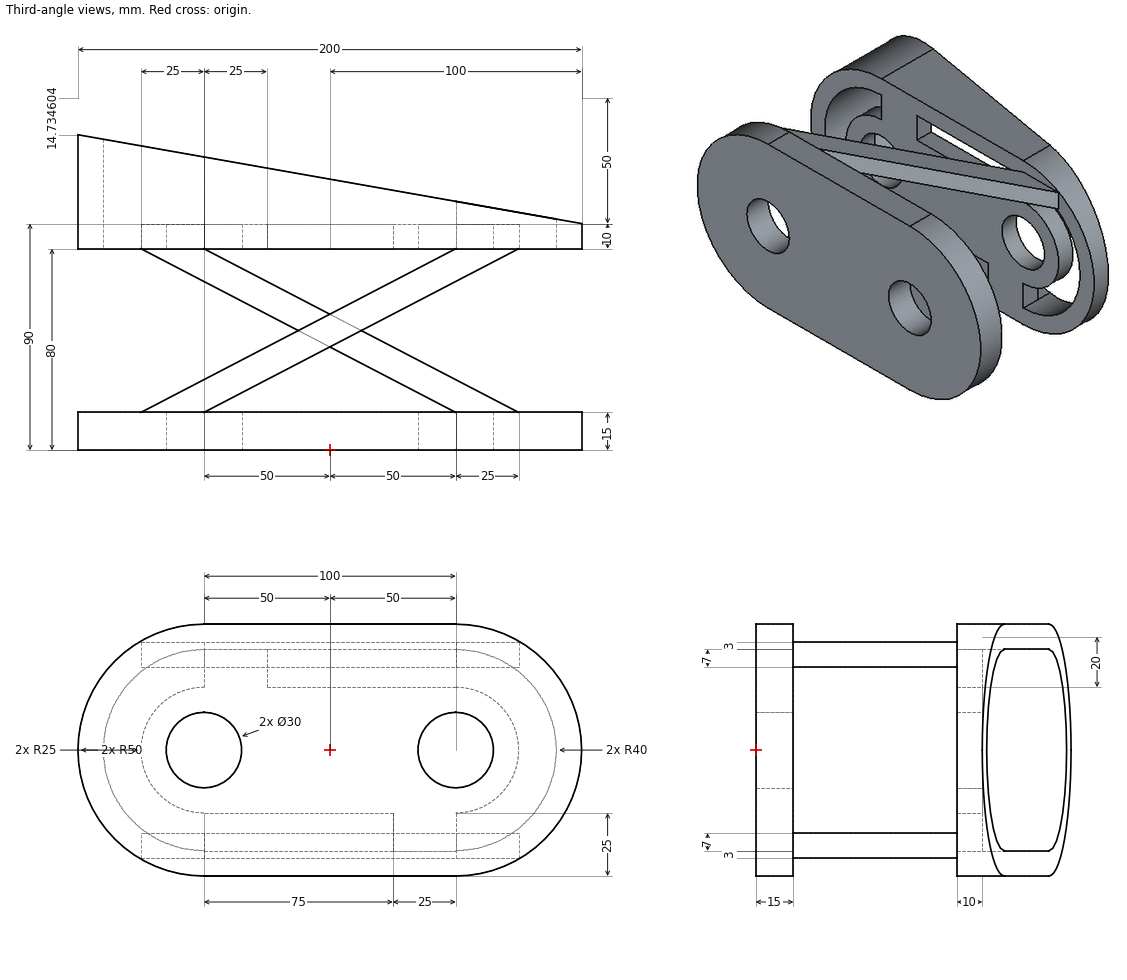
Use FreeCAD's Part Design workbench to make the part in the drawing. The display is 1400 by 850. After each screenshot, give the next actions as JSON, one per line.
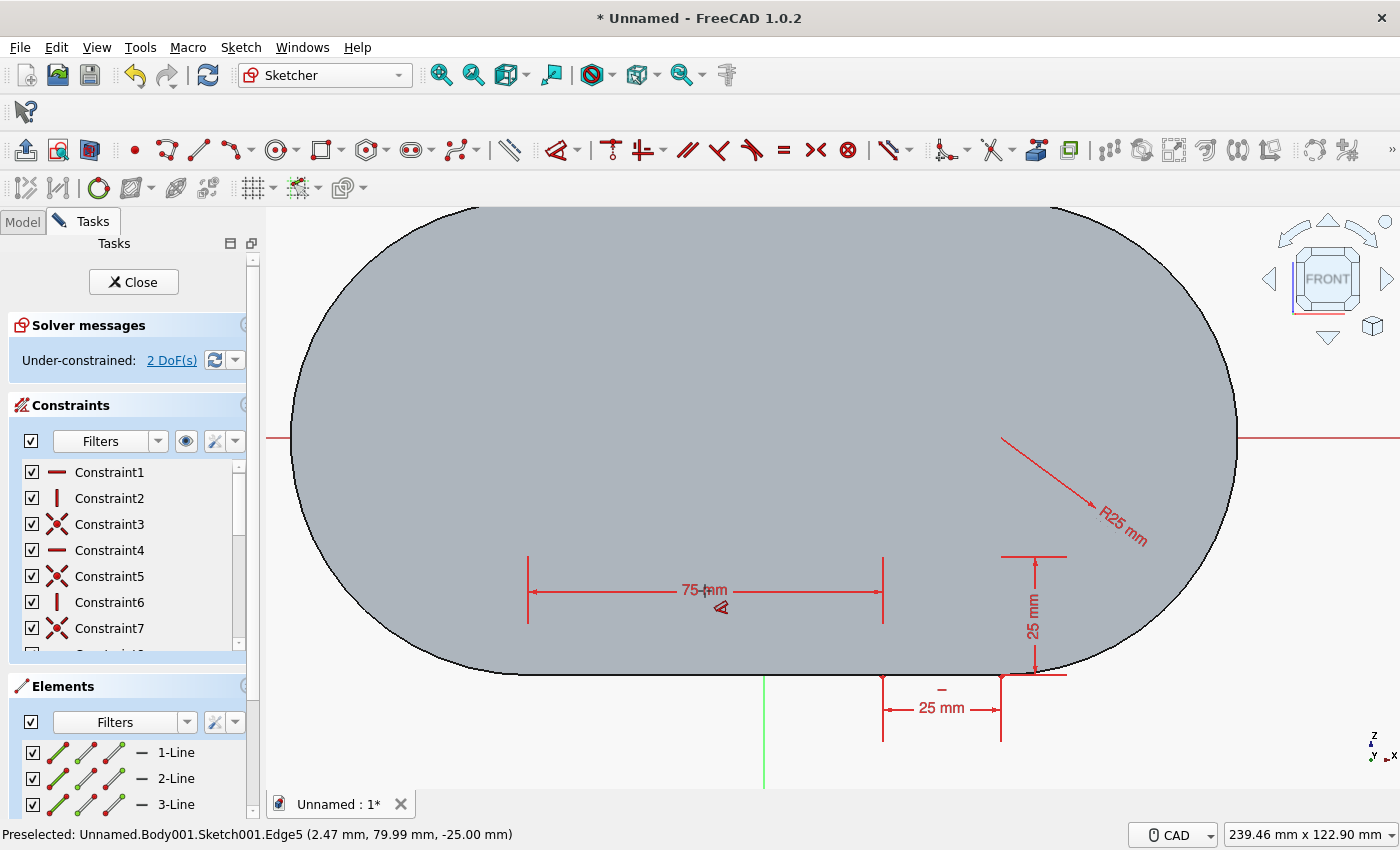
{"action": "left_click", "coordinate": [670, 320]}
{"action": "left_click", "coordinate": [656, 286]}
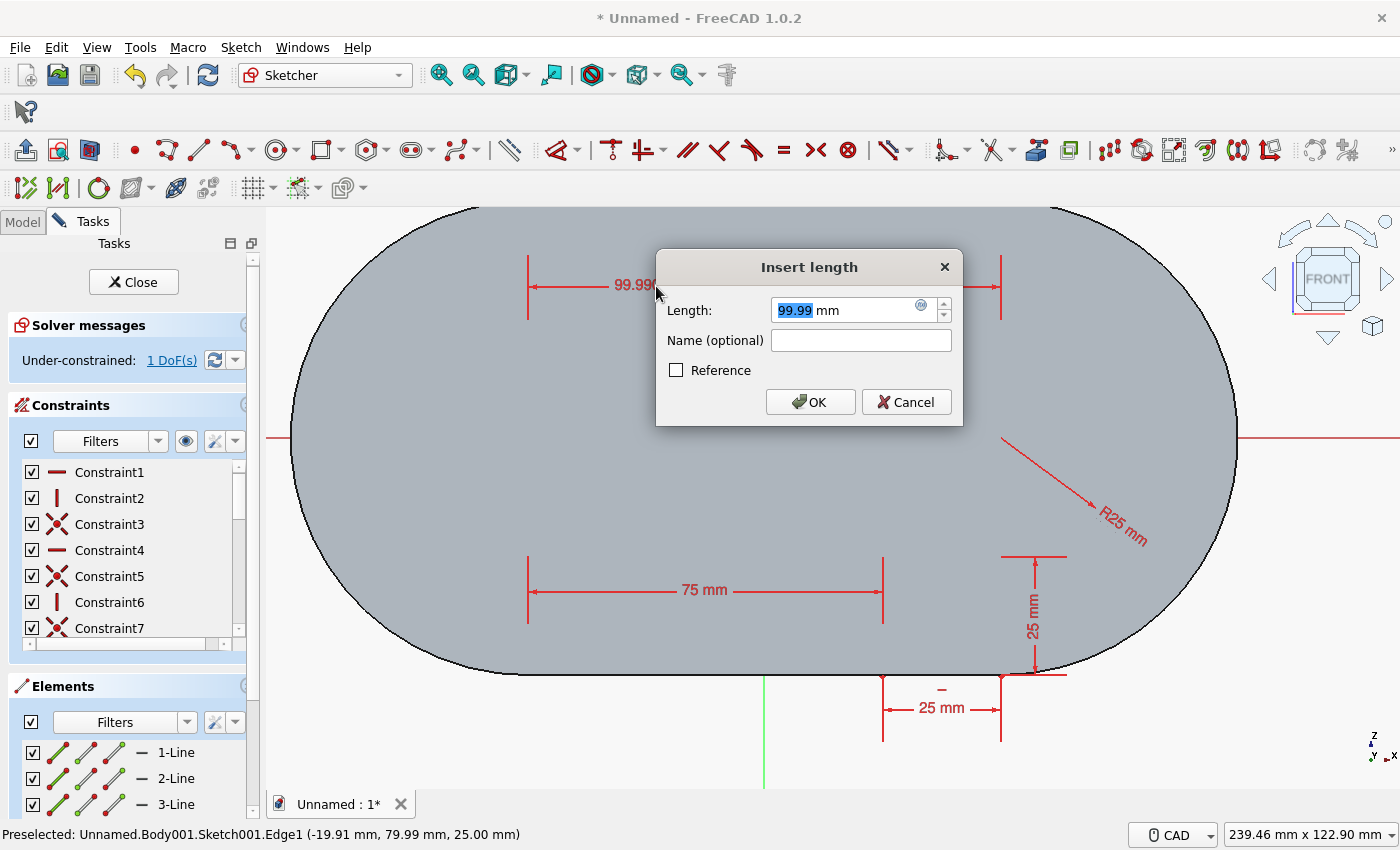
{"action": "type", "text": "100"}
{"action": "key", "text": "Return"}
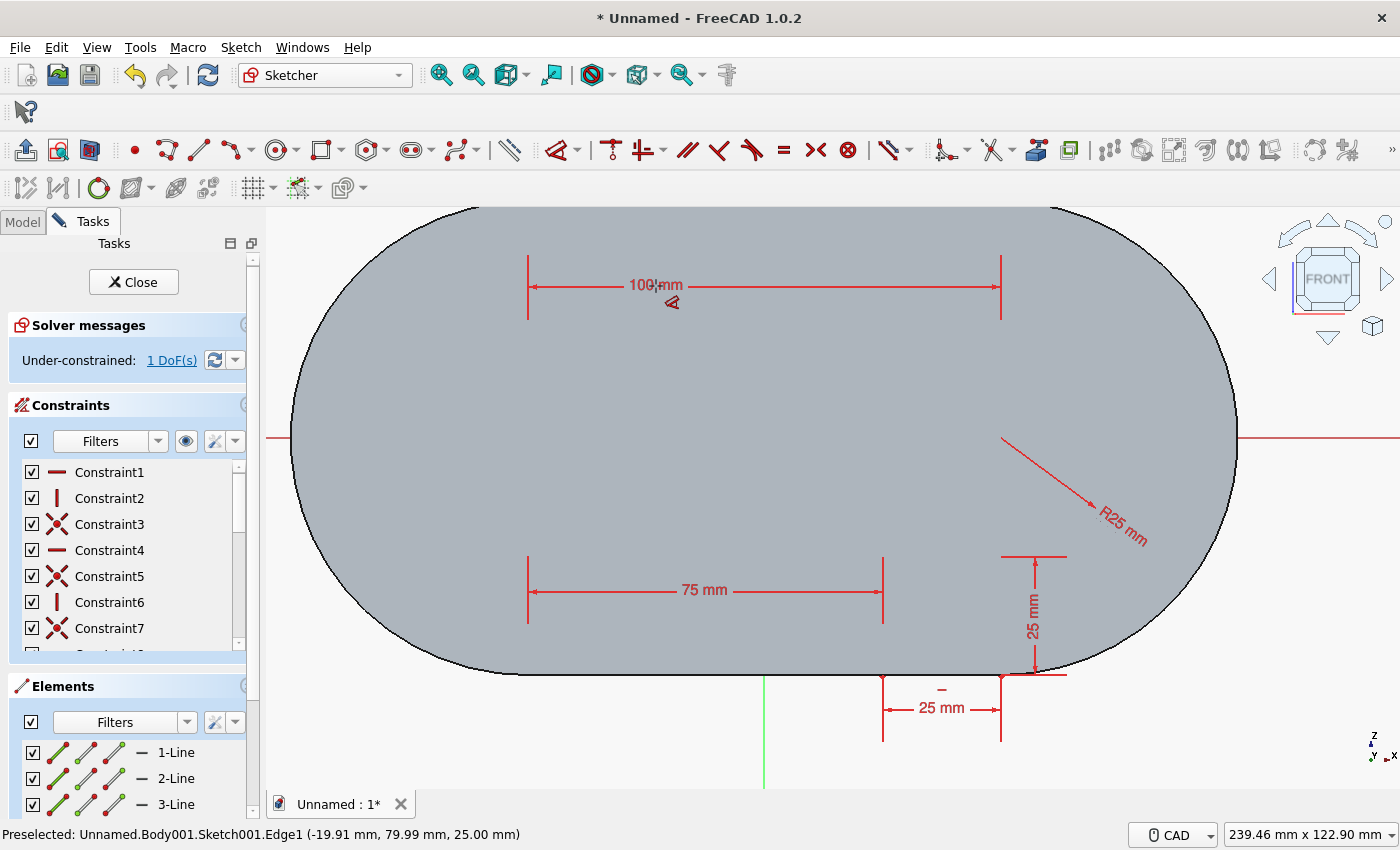
{"action": "left_click", "coordinate": [528, 320]}
{"action": "left_click", "coordinate": [563, 286]}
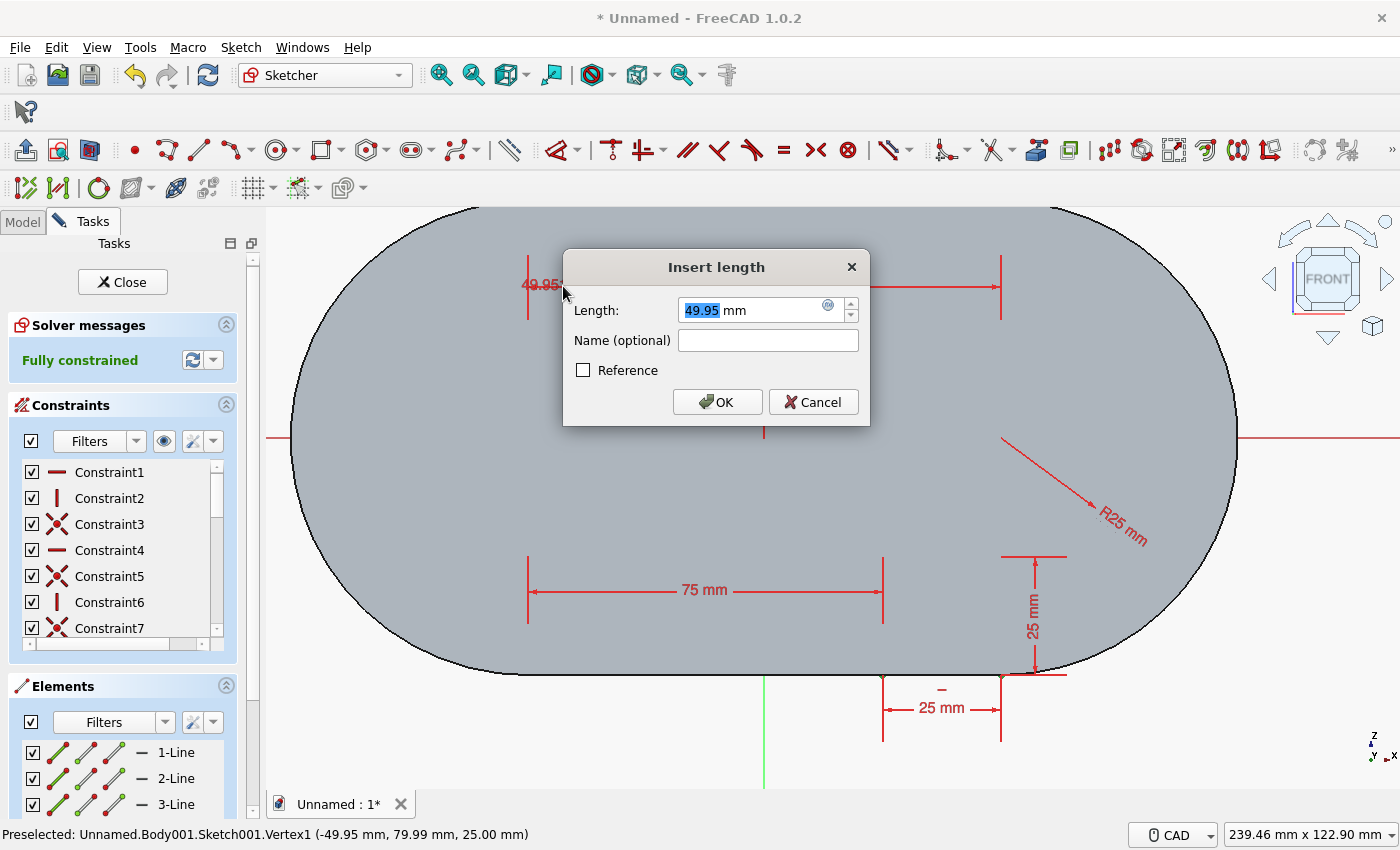
{"action": "type", "text": "50"}
{"action": "key", "text": "Return"}
{"action": "key", "text": "Escape"}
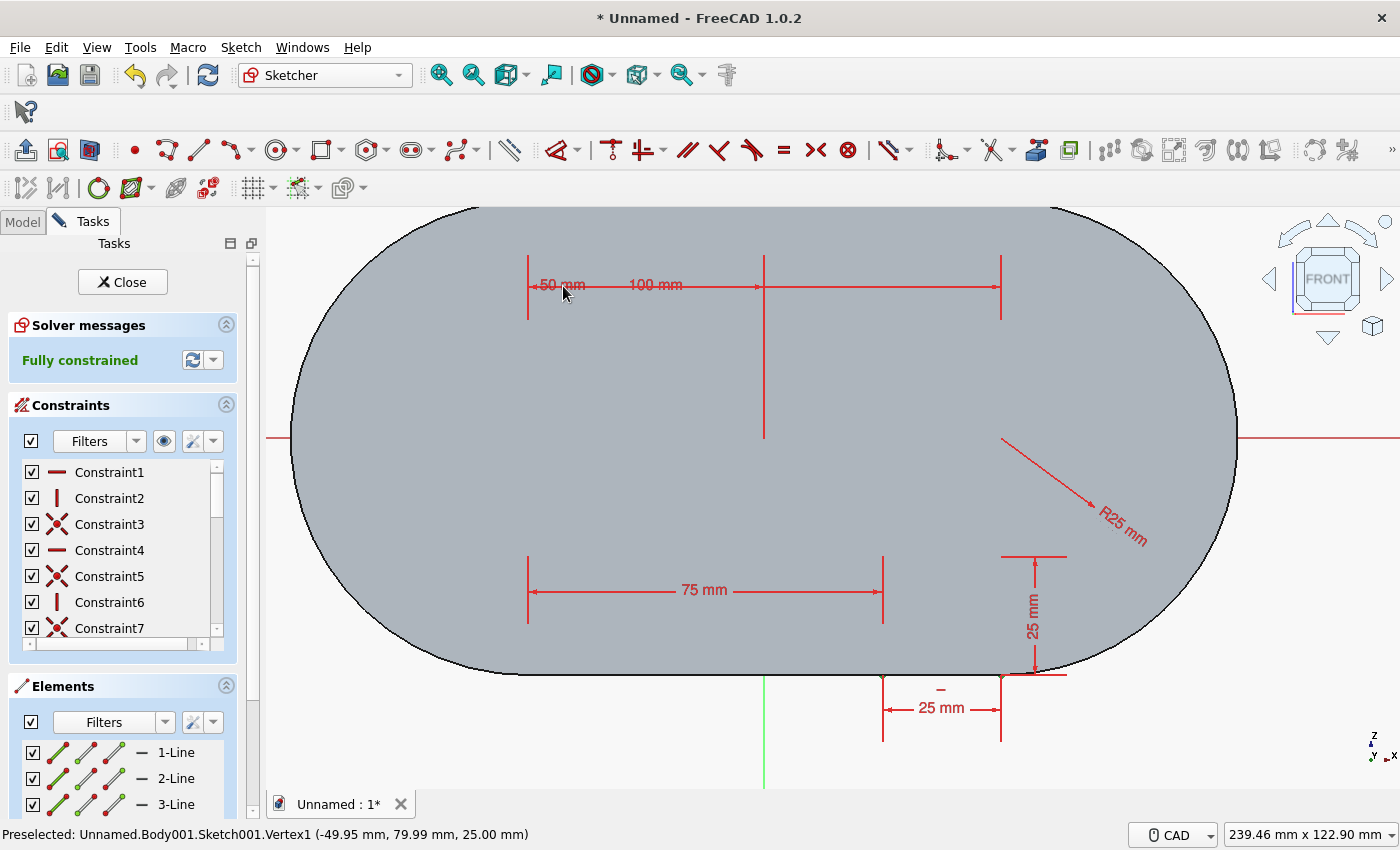
{"action": "left_click", "coordinate": [123, 282]}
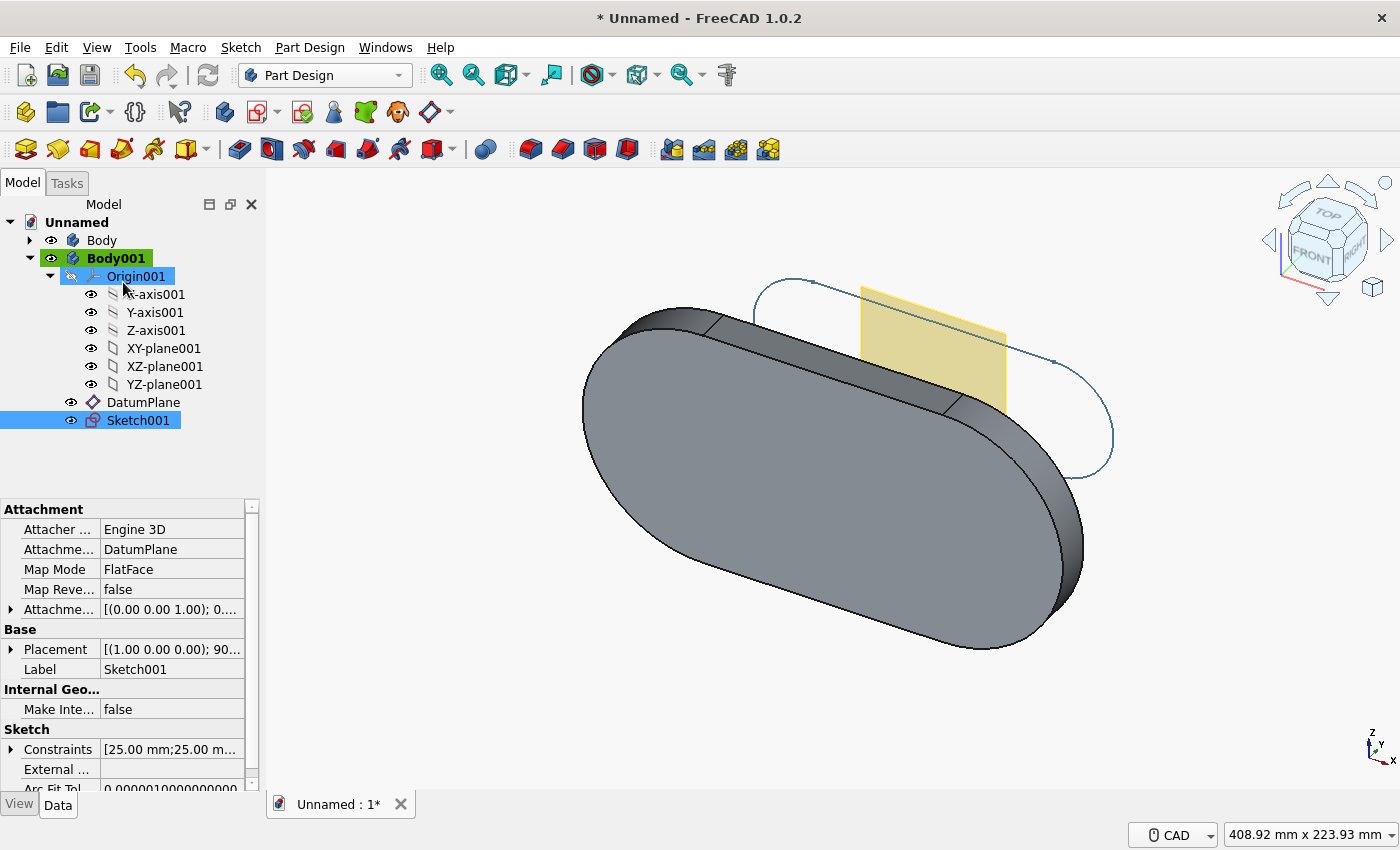
{"action": "left_click", "coordinate": [26, 150]}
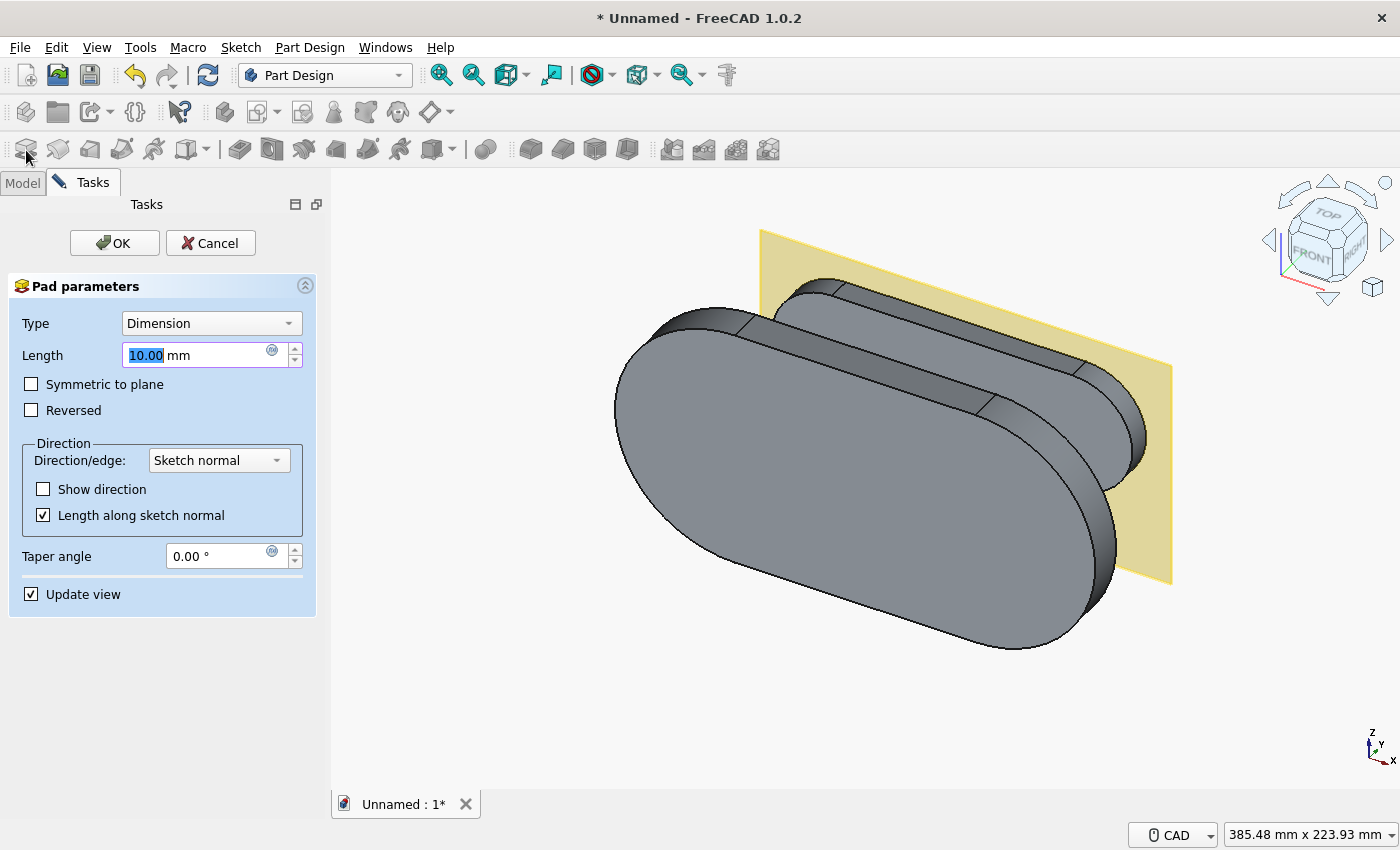
{"action": "type", "text": "10"}
{"action": "key", "text": "Tab"}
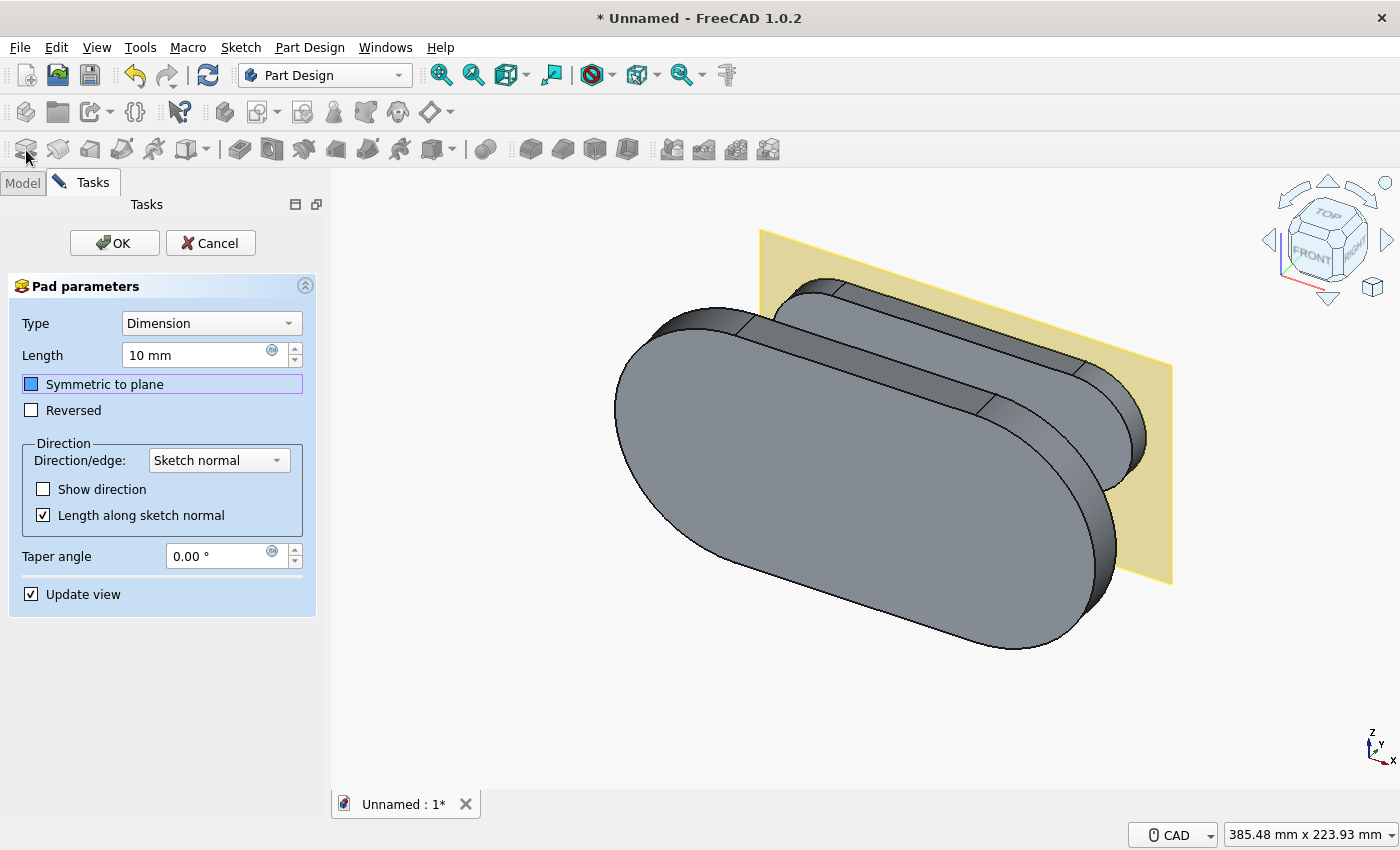
{"action": "left_click", "coordinate": [30, 410]}